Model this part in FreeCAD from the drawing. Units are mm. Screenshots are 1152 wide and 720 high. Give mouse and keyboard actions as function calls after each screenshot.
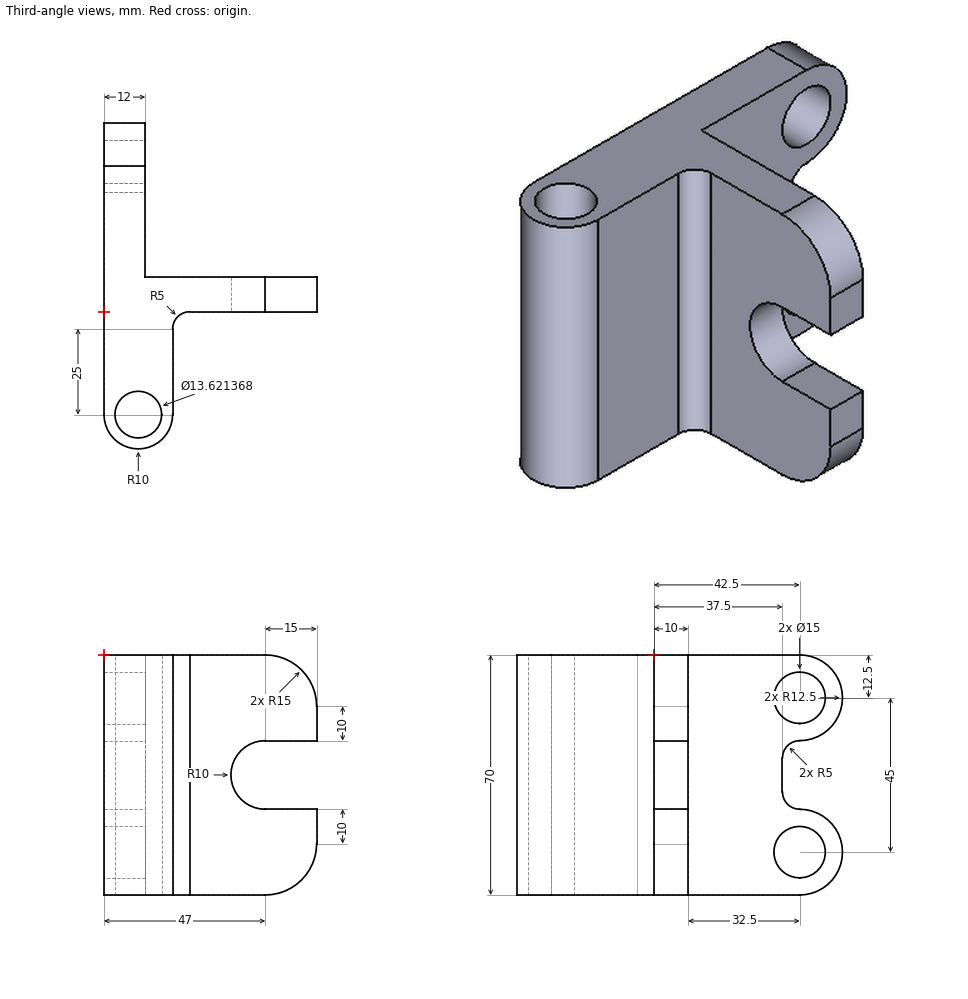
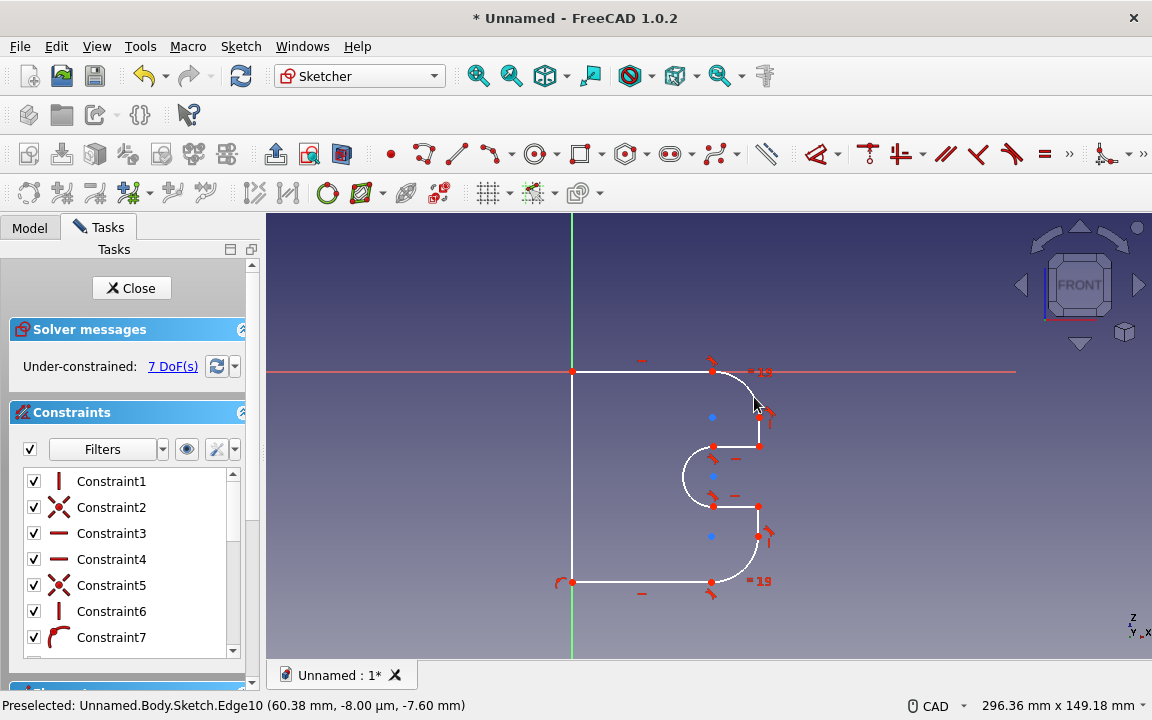
click(816, 154)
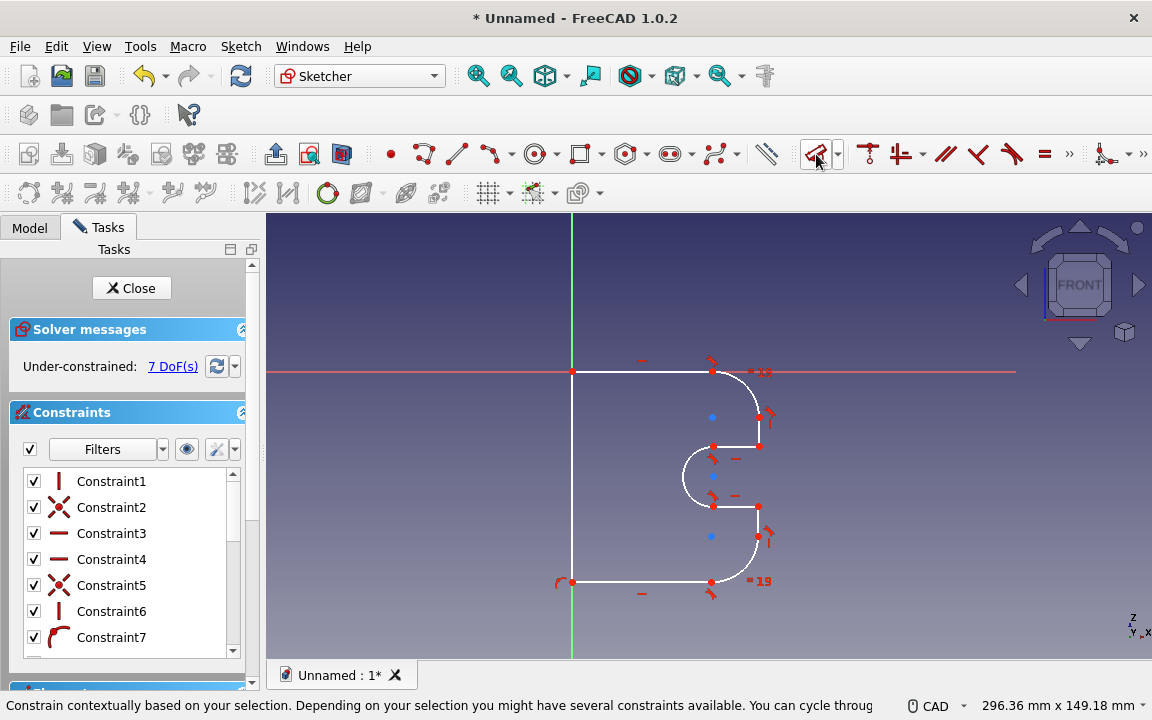
scroll(689, 459, up, 2)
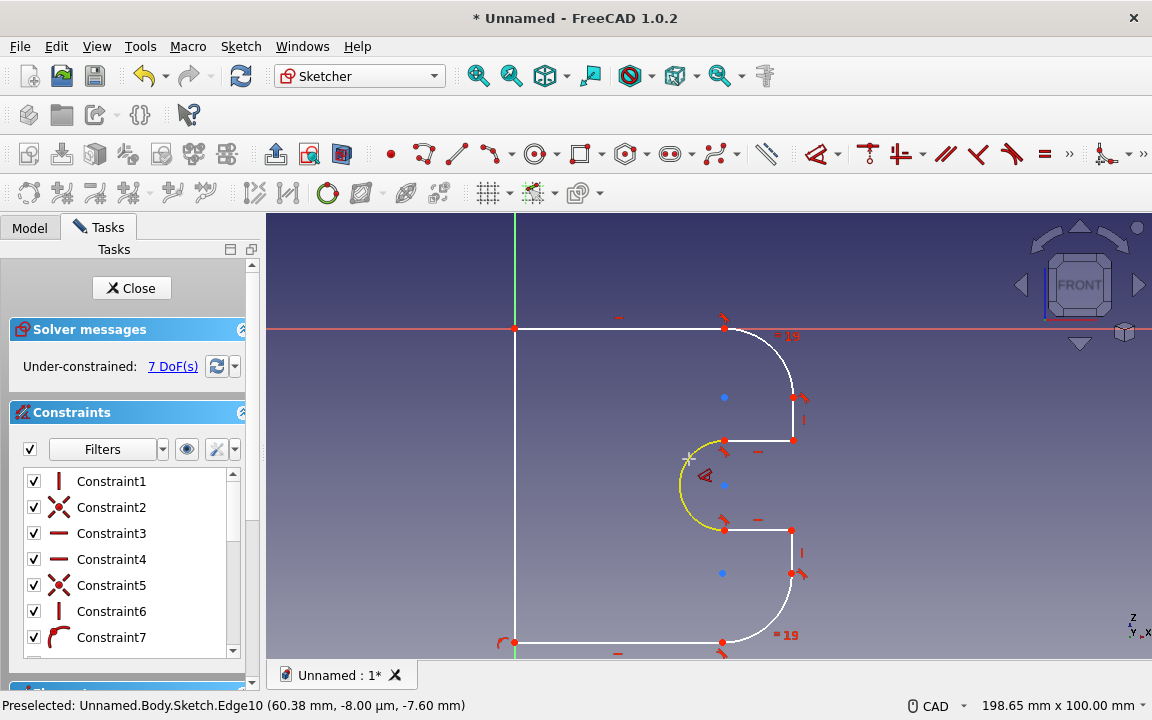
click(688, 459)
click(662, 440)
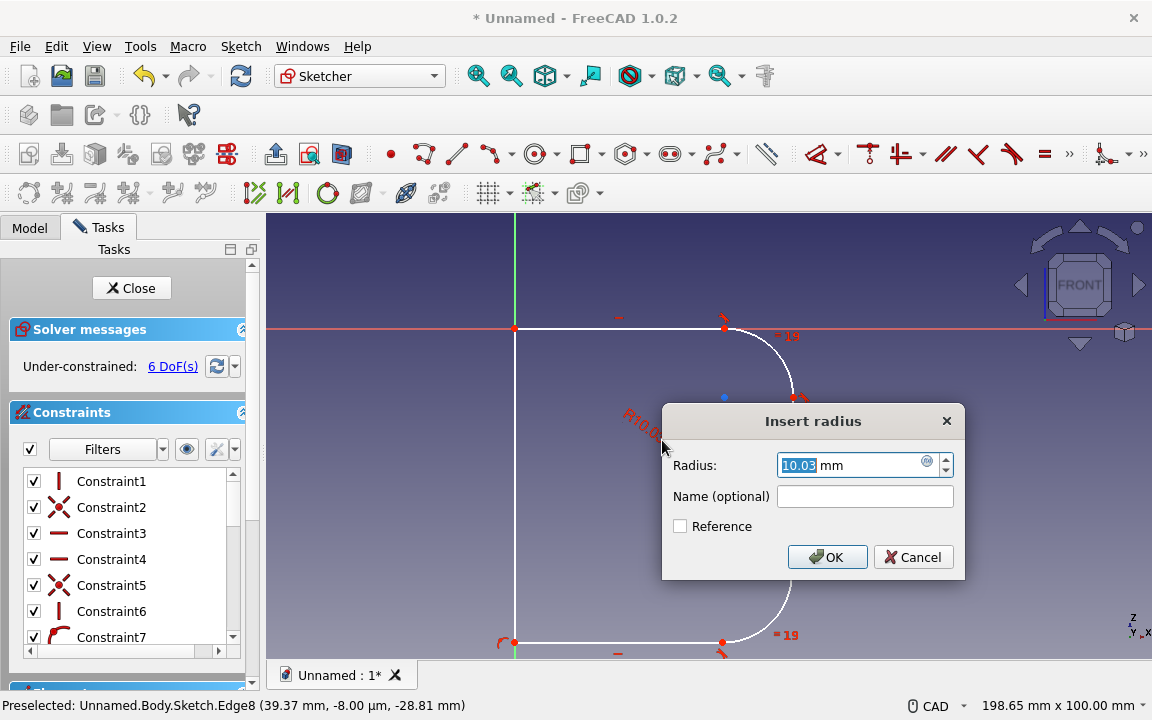
text(10)
key(Return)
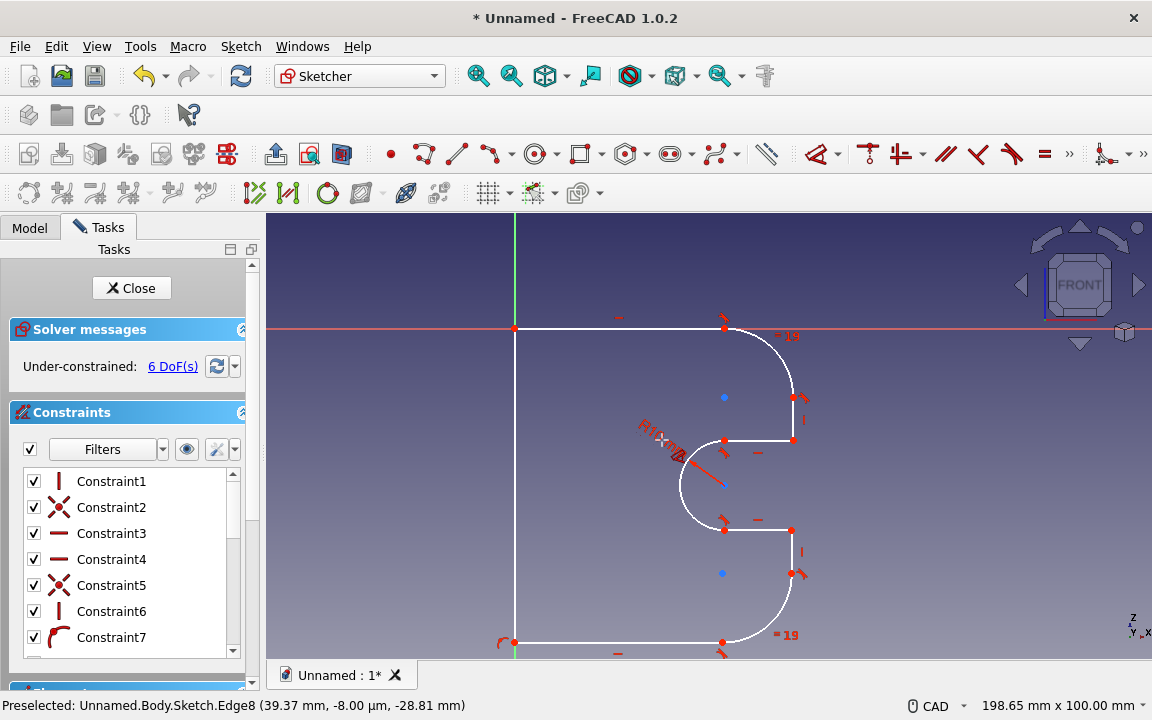
click(784, 605)
click(812, 620)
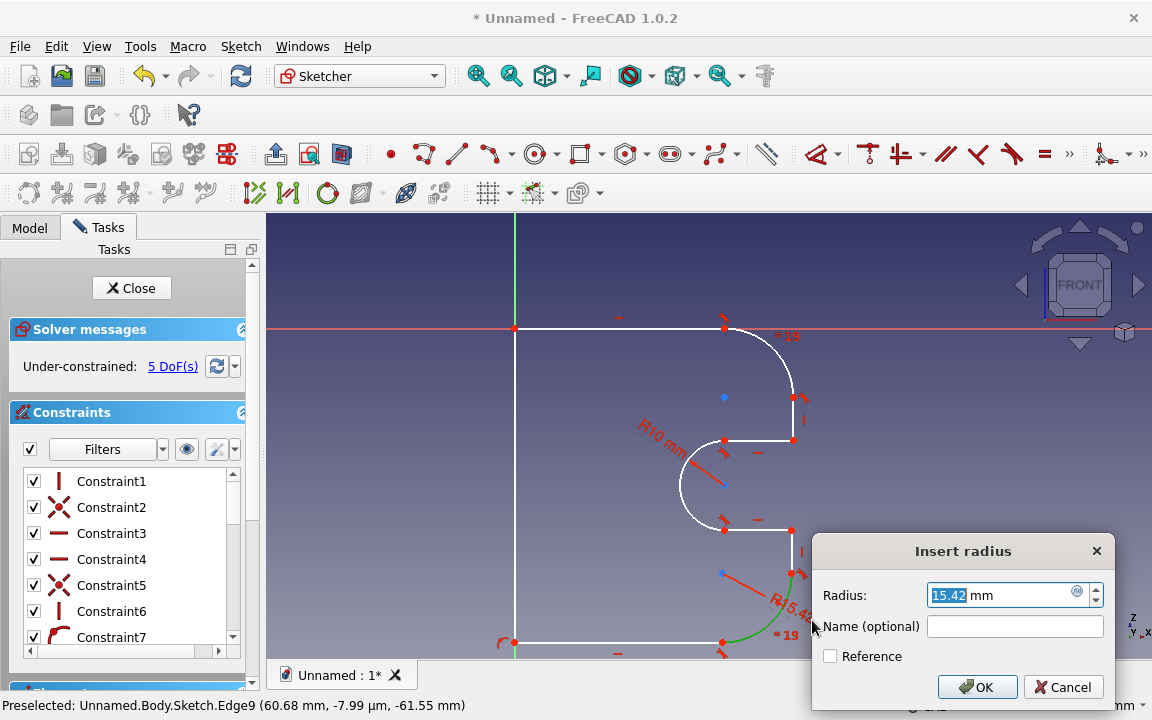
text(15)
key(Return)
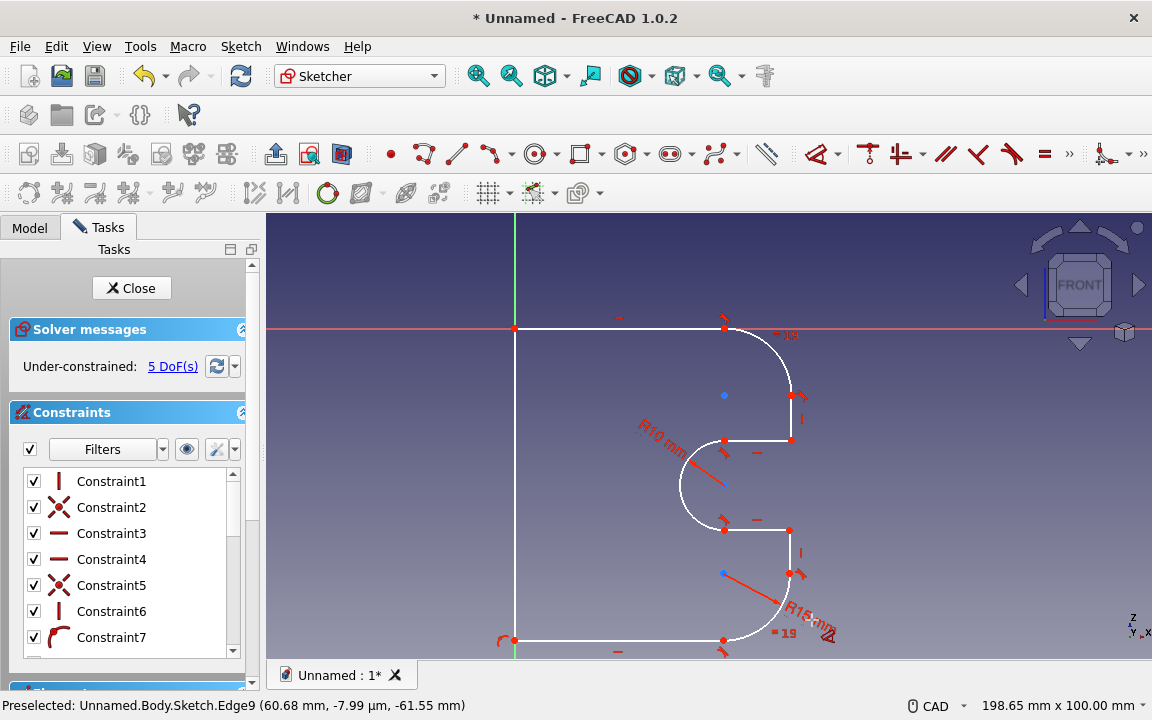
click(791, 409)
click(825, 418)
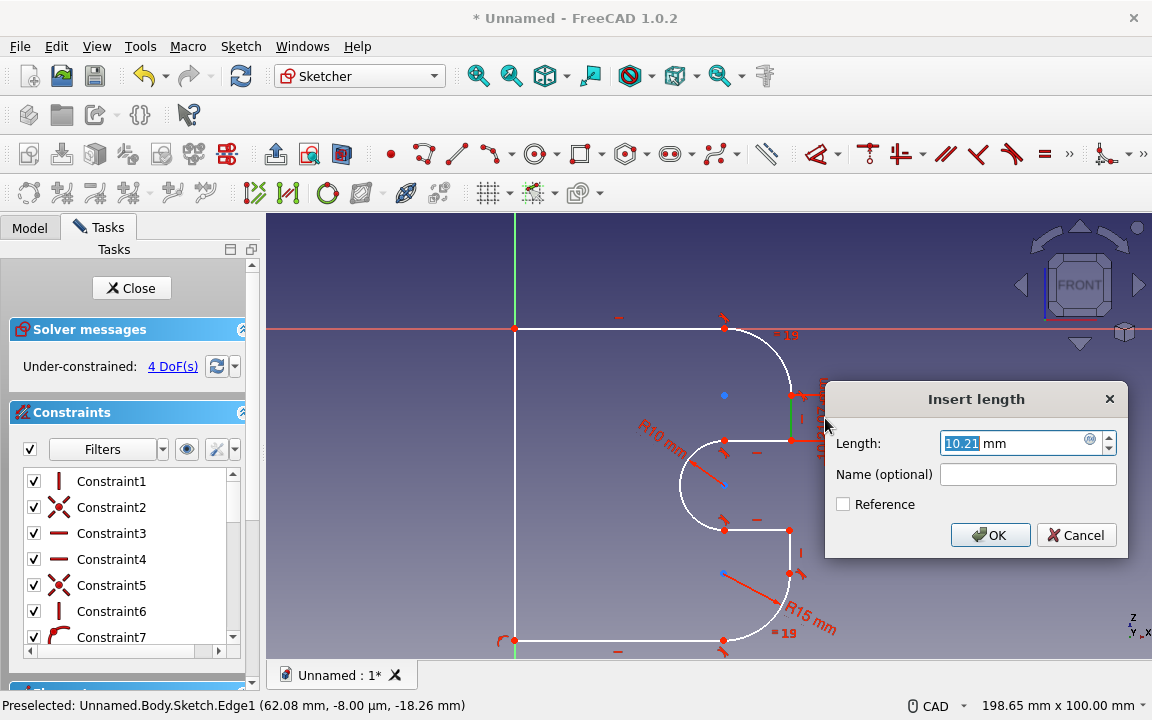
text(10)
key(Return)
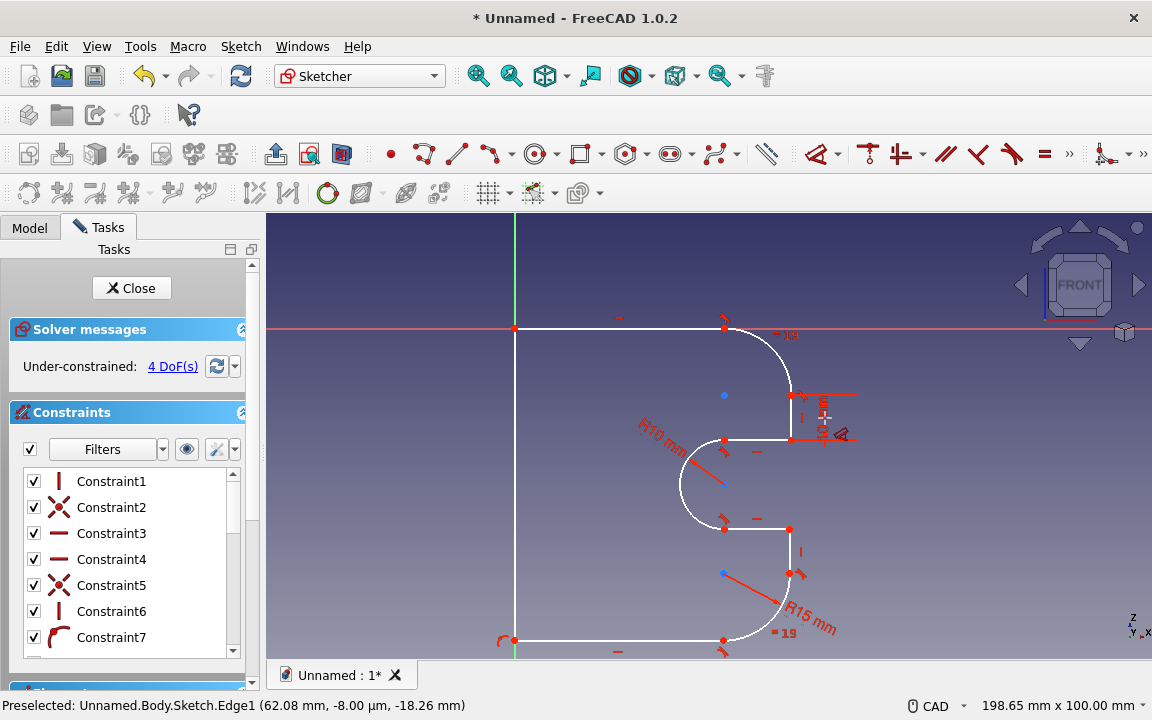
click(771, 440)
click(743, 406)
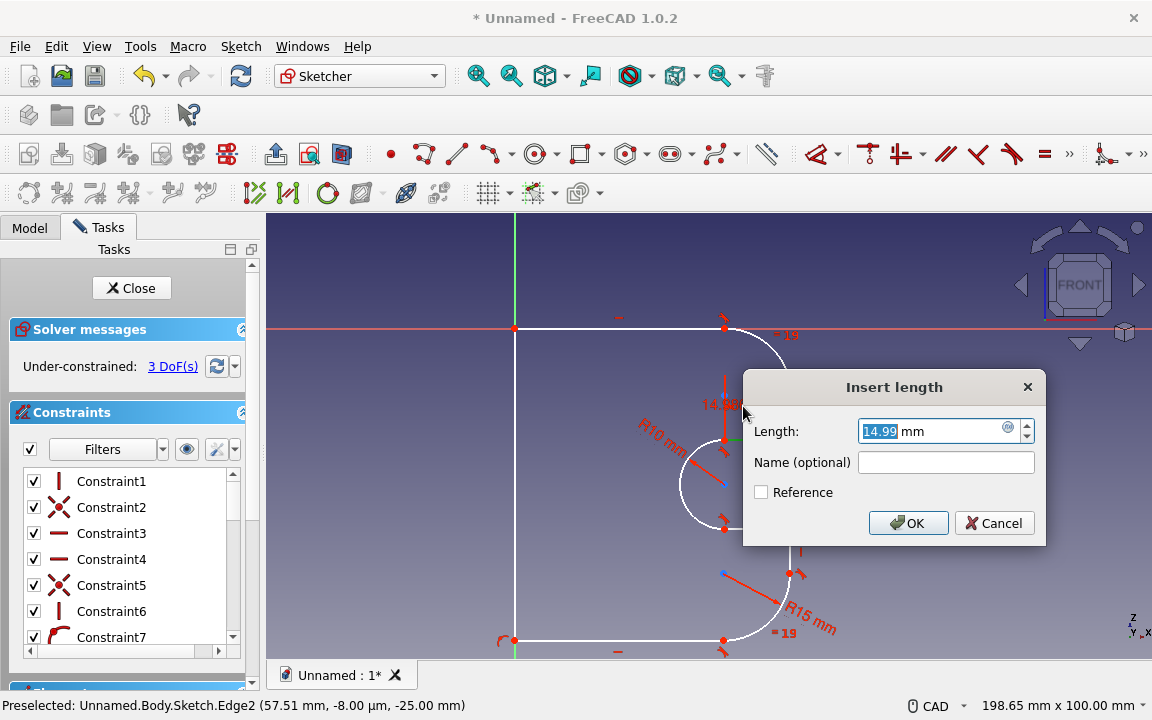
text(15)
key(Return)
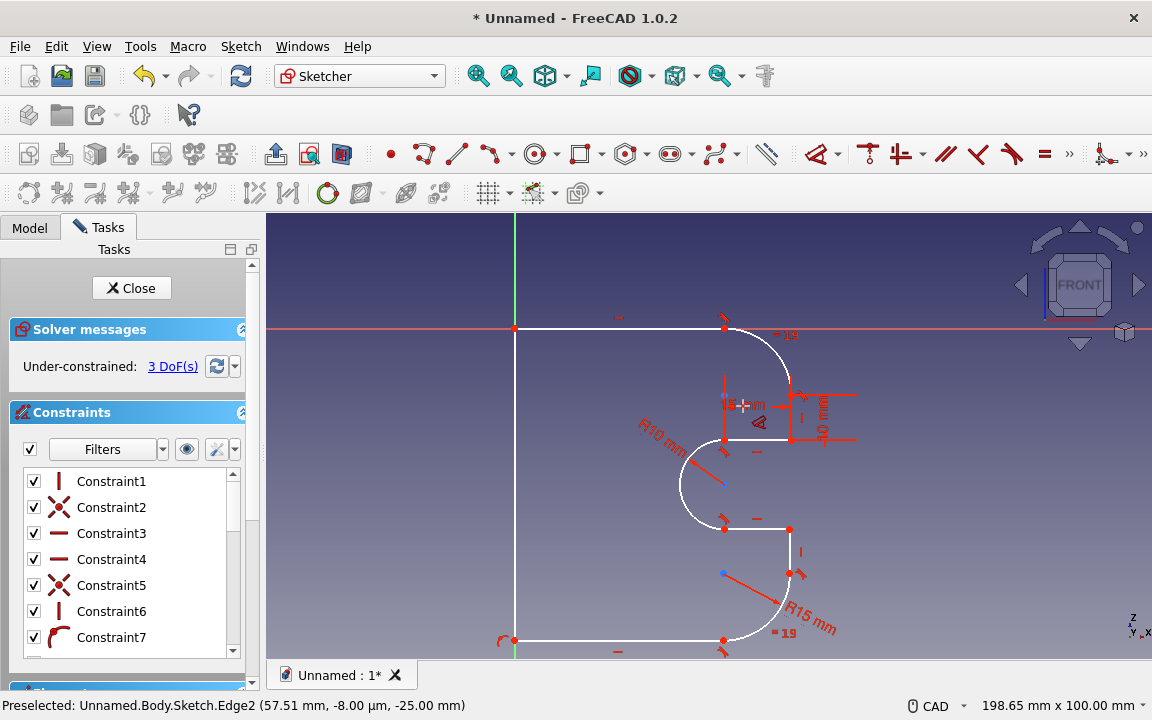
click(744, 529)
click(757, 563)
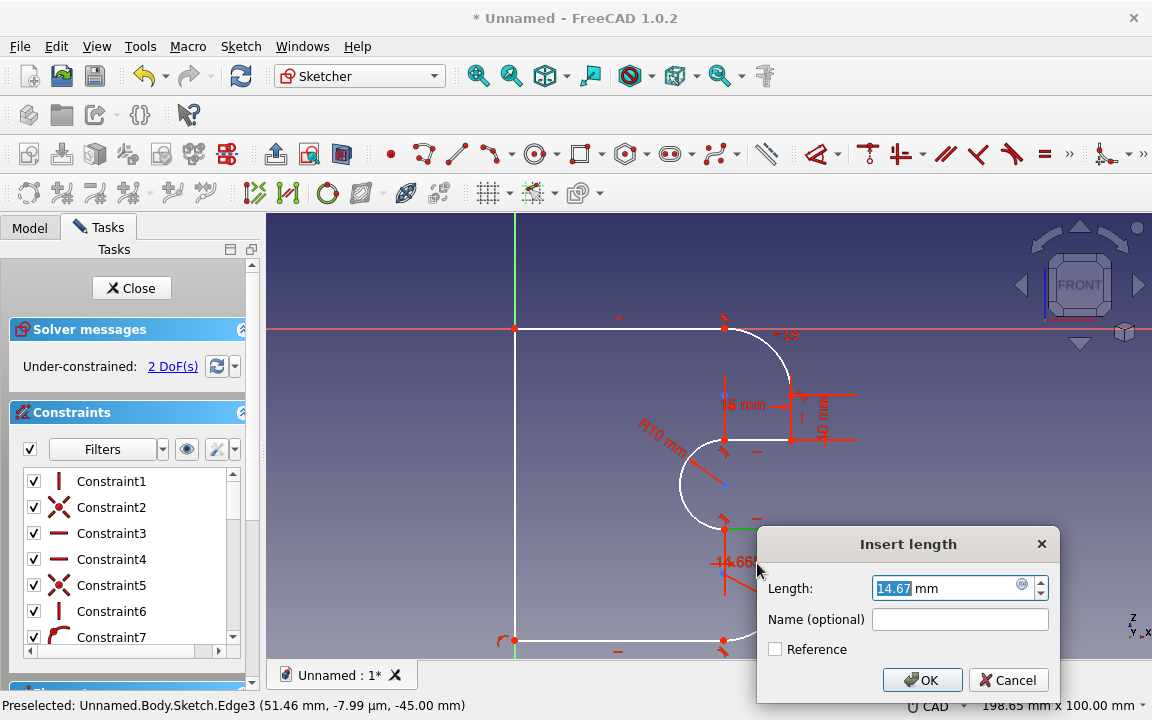
text(15)
key(Return)